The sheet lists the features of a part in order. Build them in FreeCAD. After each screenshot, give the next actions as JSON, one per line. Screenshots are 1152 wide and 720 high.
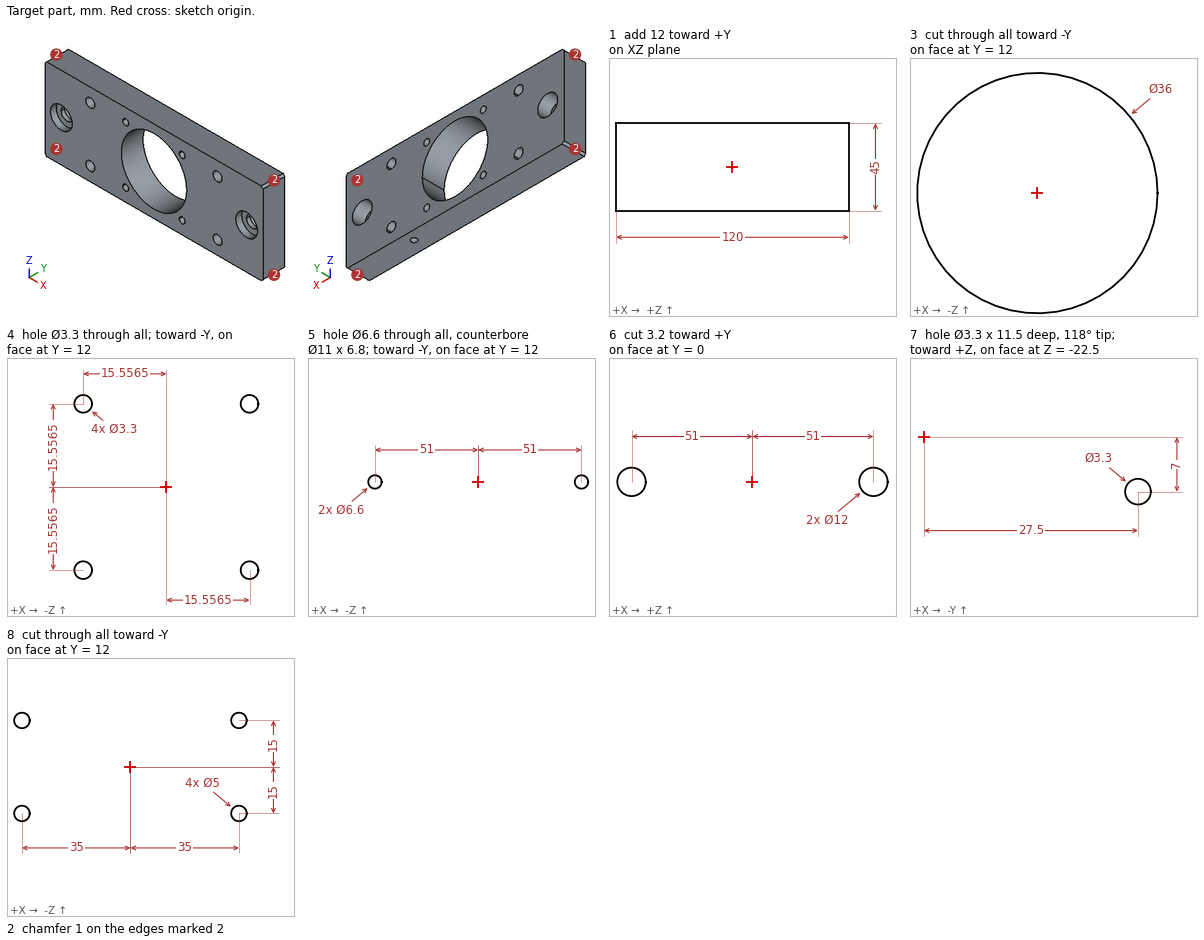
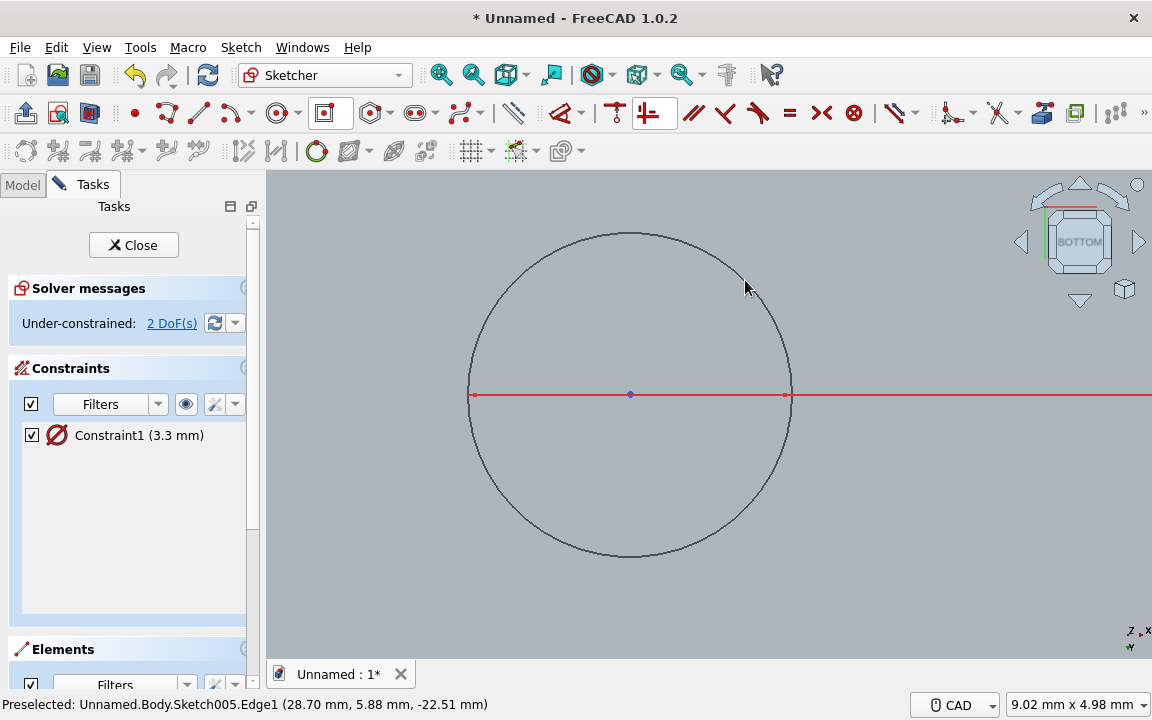
{"action": "left_click", "coordinate": [560, 114]}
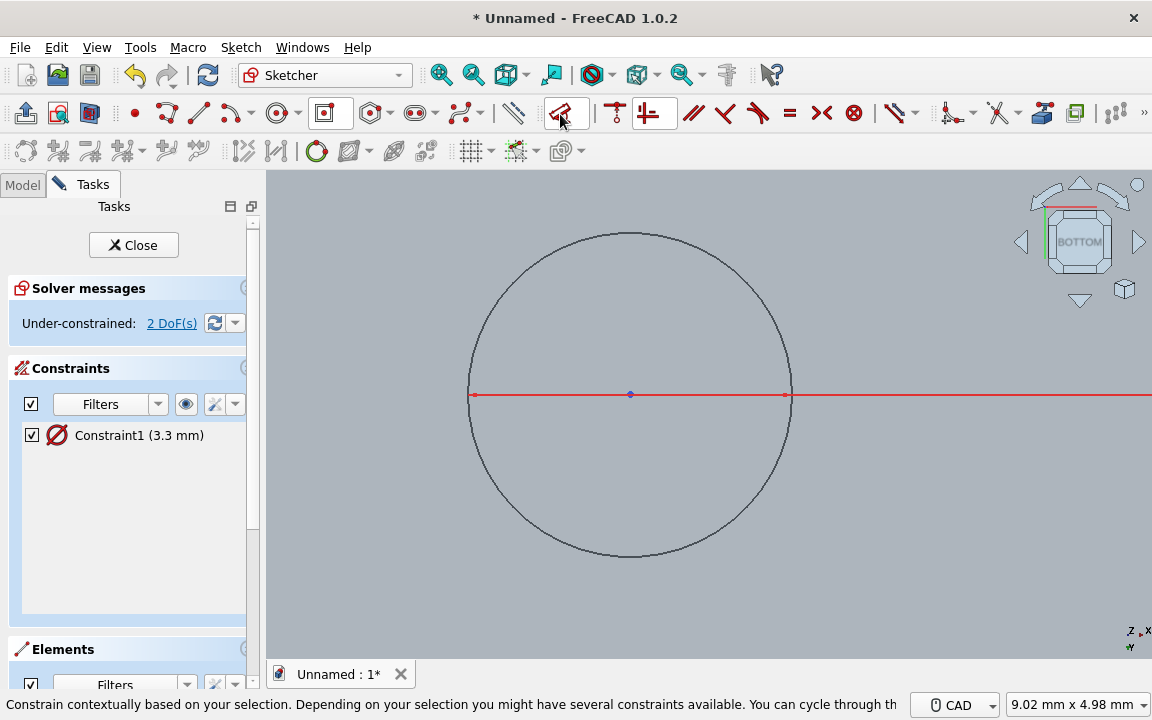
{"action": "left_click", "coordinate": [630, 395]}
{"action": "left_click", "coordinate": [664, 297]}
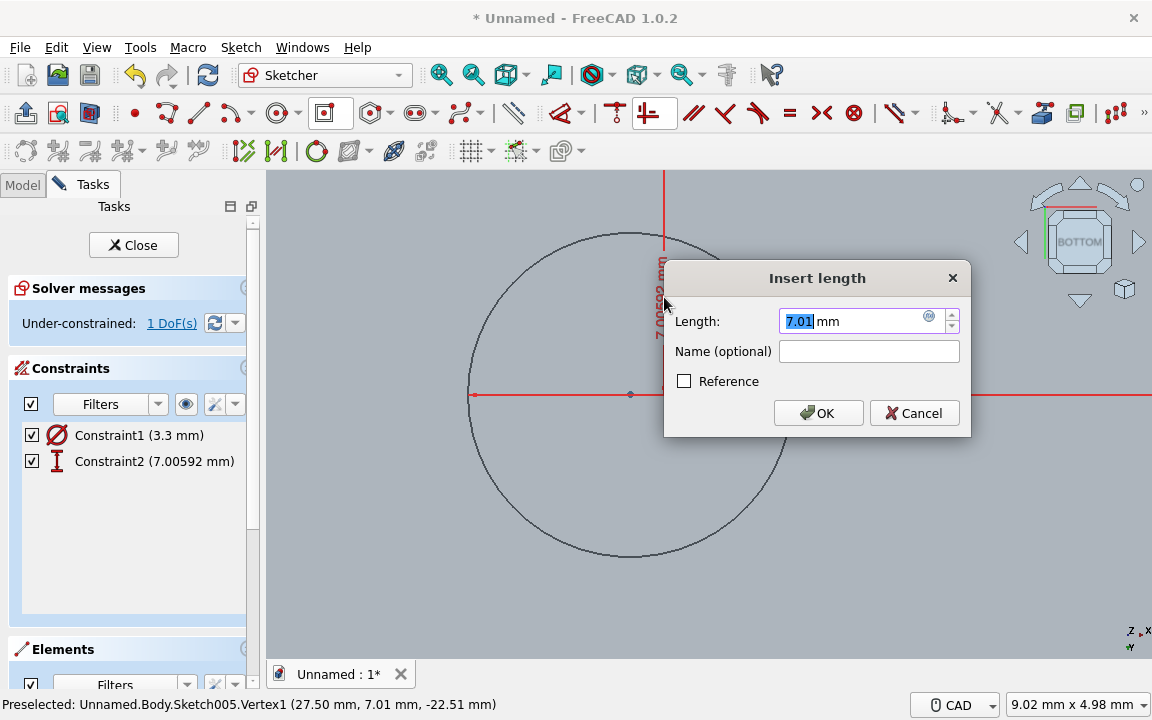
{"action": "type", "text": "7"}
{"action": "key", "text": "Return"}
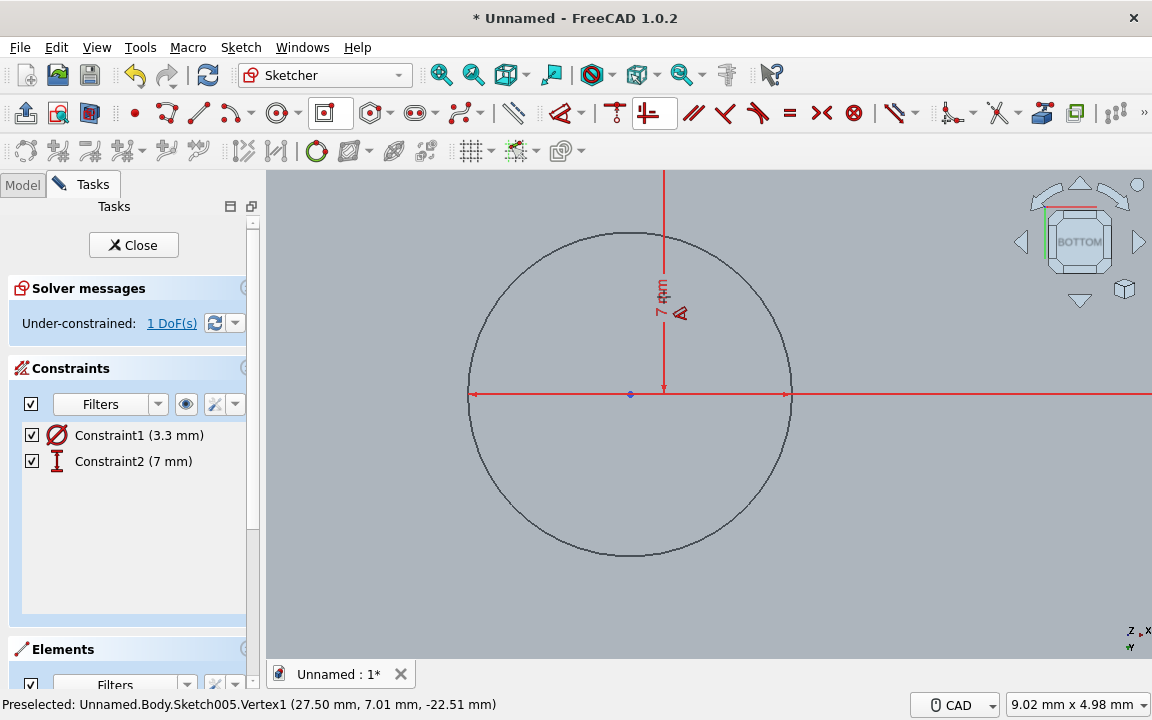
{"action": "left_click", "coordinate": [630, 394]}
{"action": "left_click", "coordinate": [385, 428]}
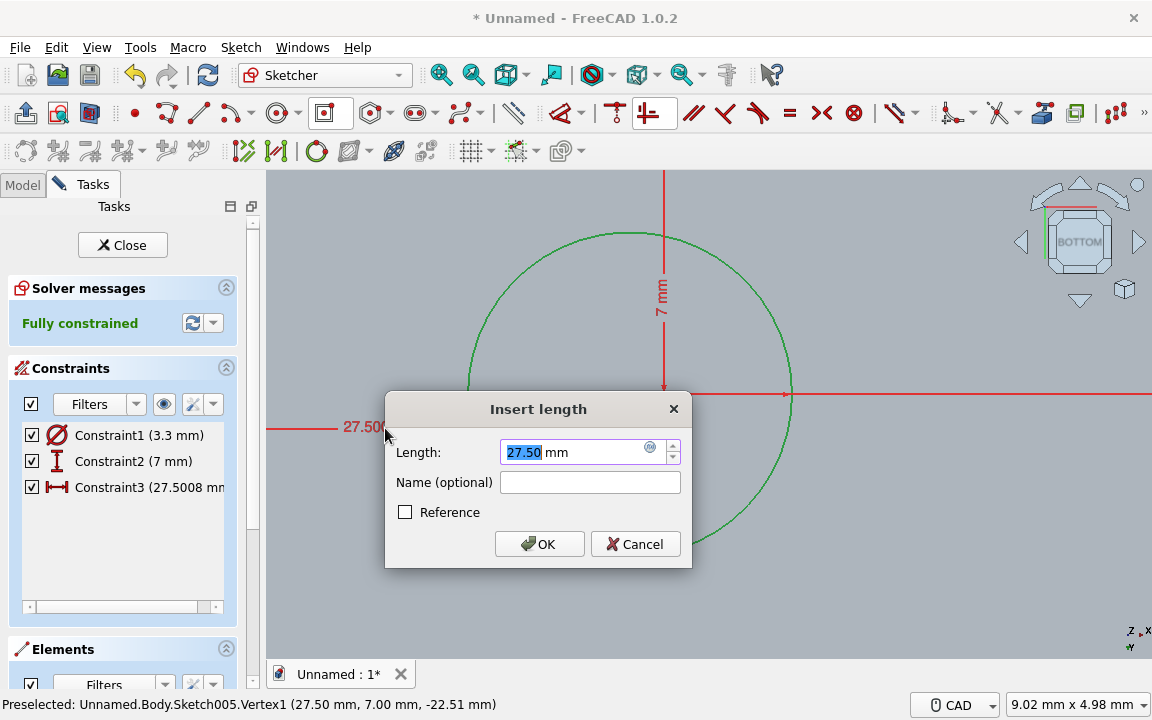
{"action": "type", "text": "27.5"}
{"action": "key", "text": "Return"}
{"action": "key", "text": "Escape"}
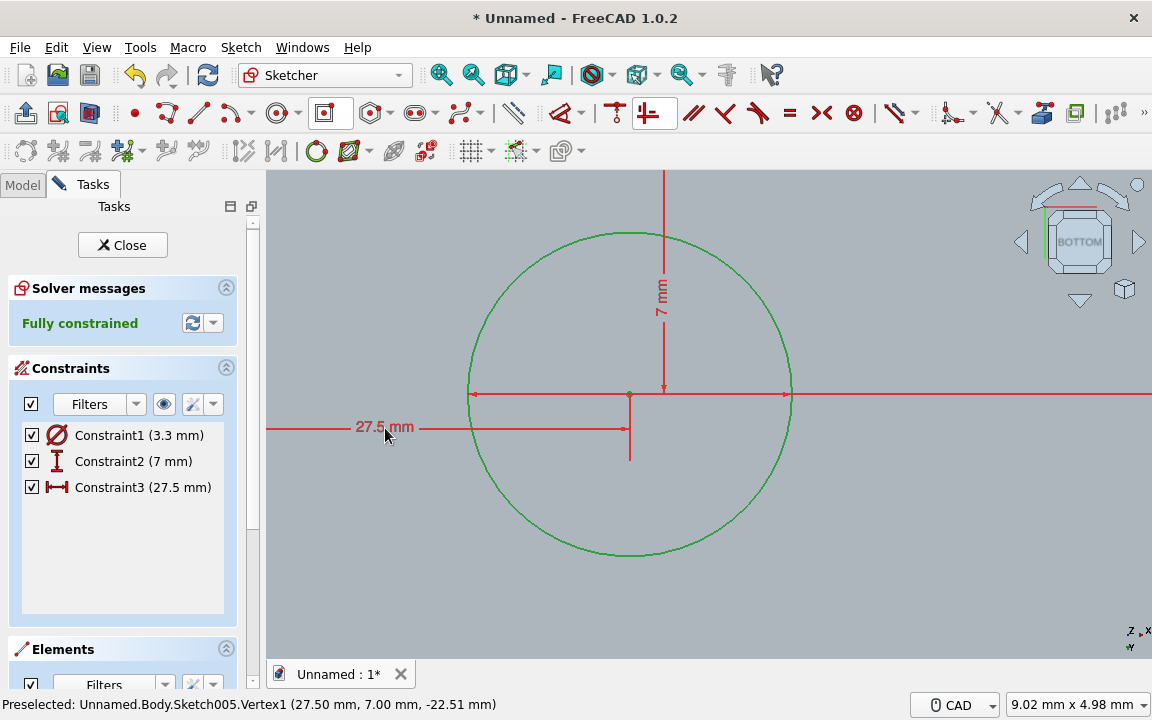
{"action": "left_click", "coordinate": [123, 245]}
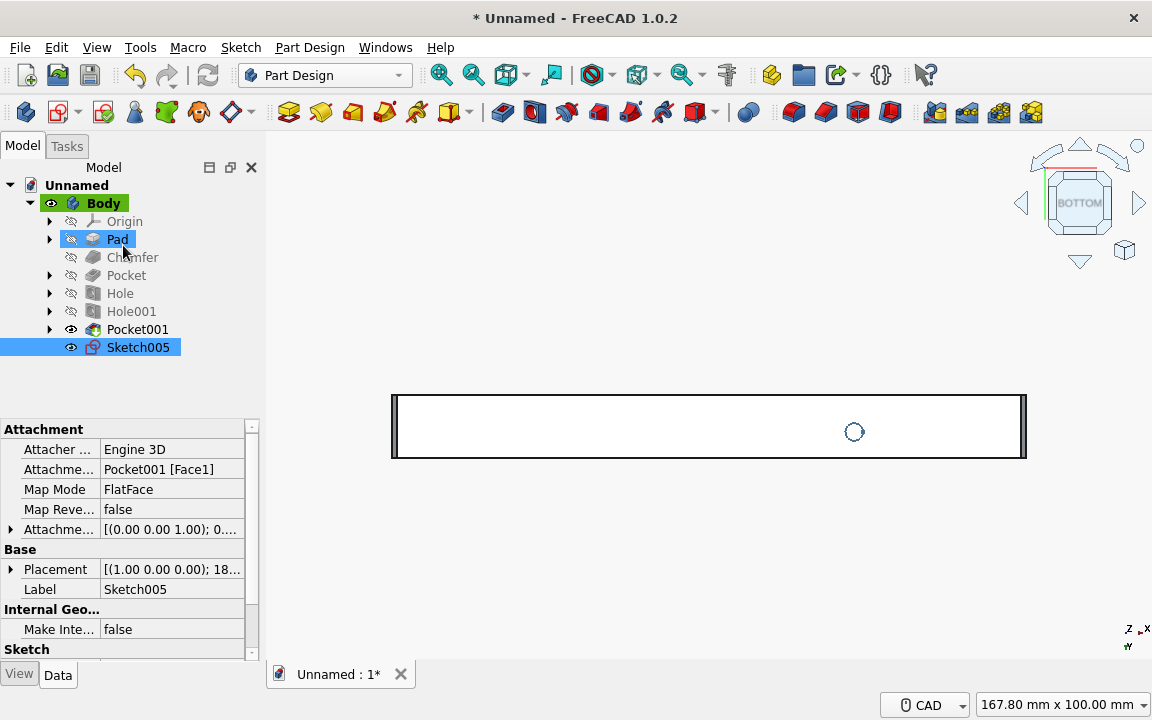
{"action": "left_click", "coordinate": [536, 112]}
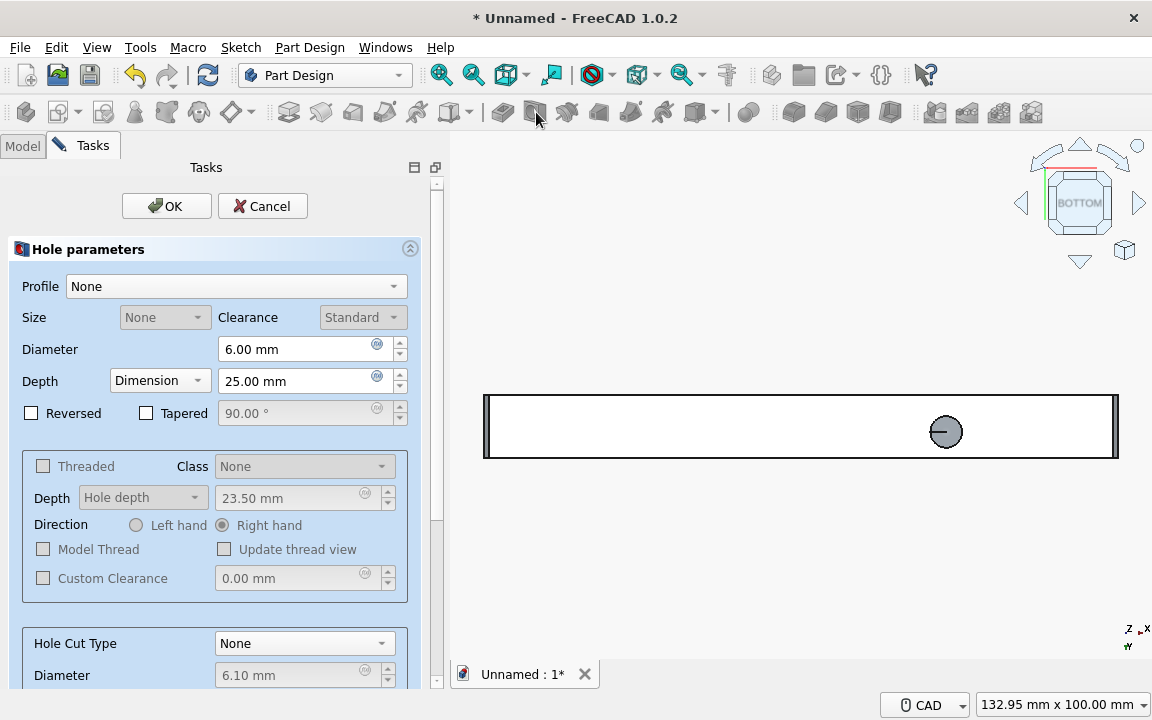
{"action": "triple_click", "coordinate": [305, 349]}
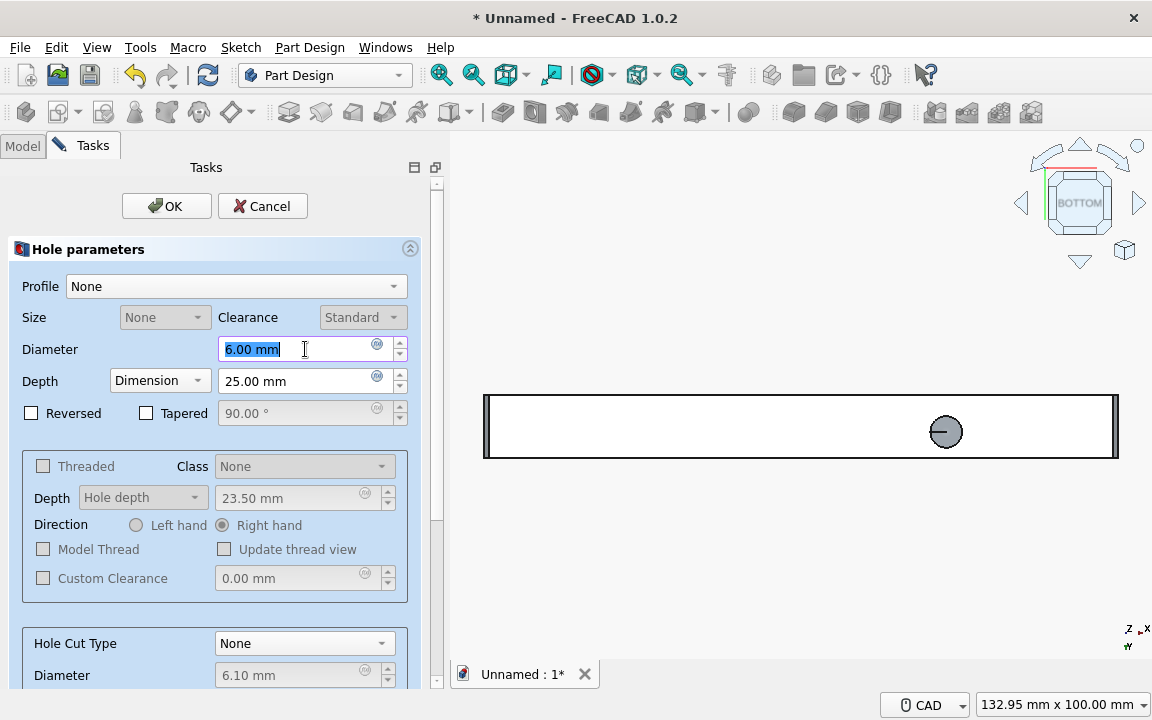
{"action": "type", "text": "3.3"}
{"action": "key", "text": "Tab"}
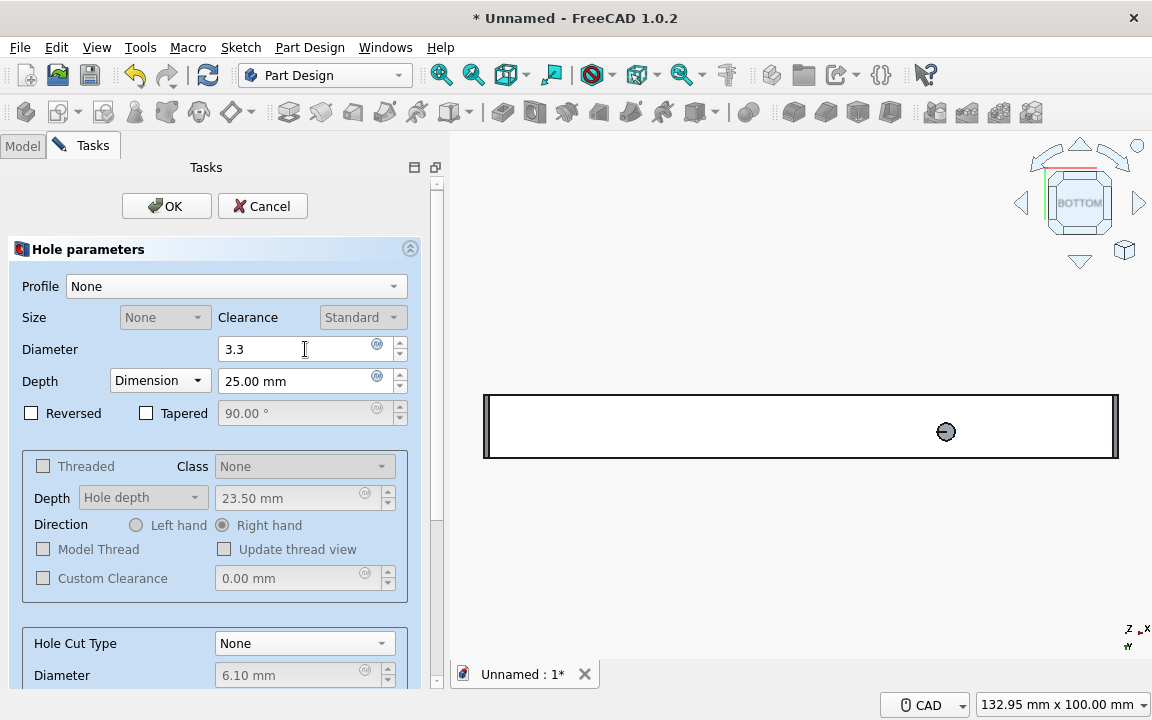
{"action": "triple_click", "coordinate": [305, 381]}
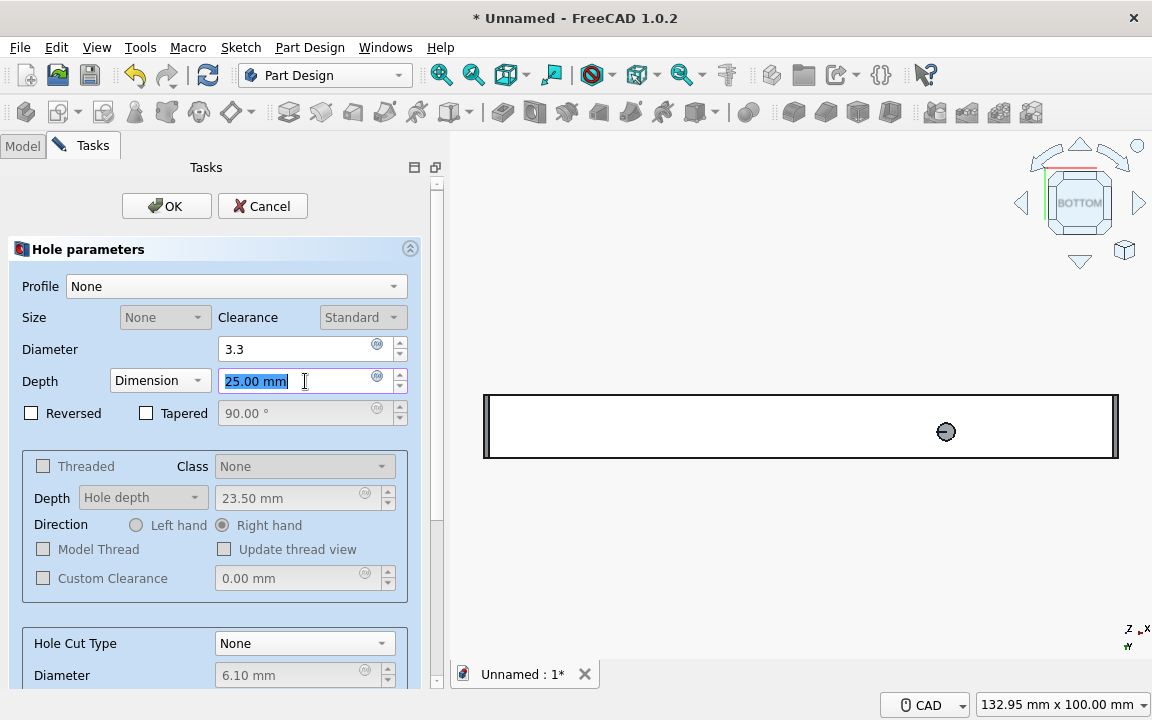
{"action": "type", "text": "11.5"}
{"action": "key", "text": "Tab"}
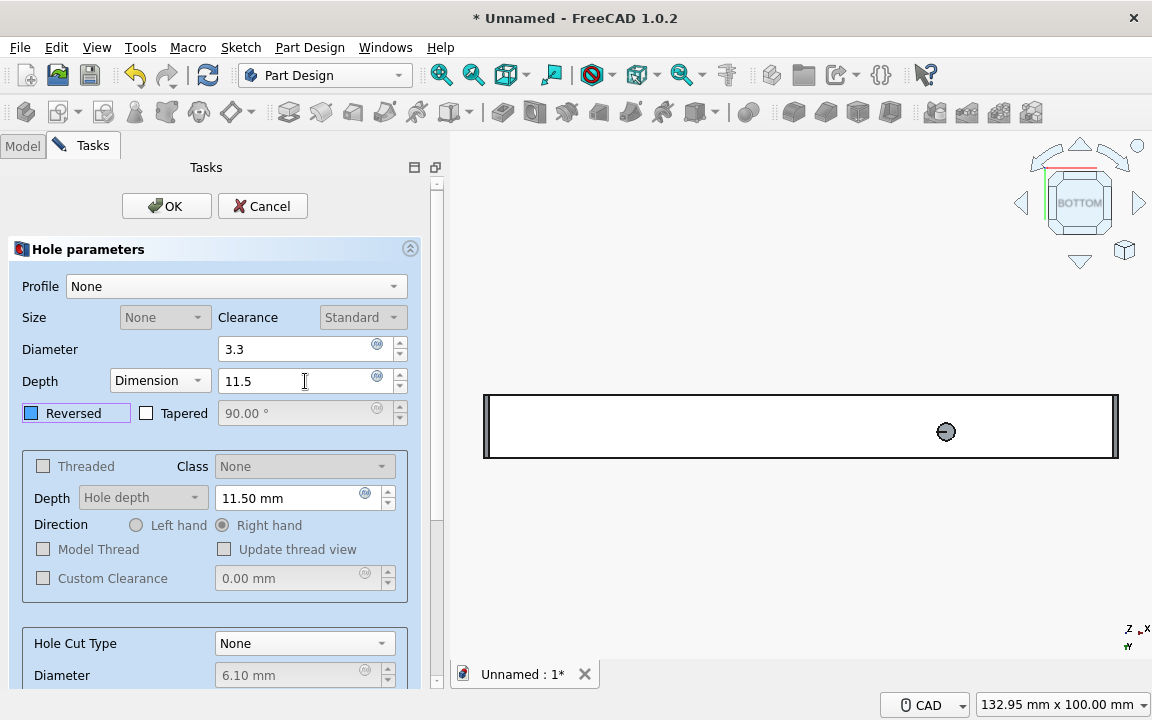
{"action": "left_click", "coordinate": [167, 206]}